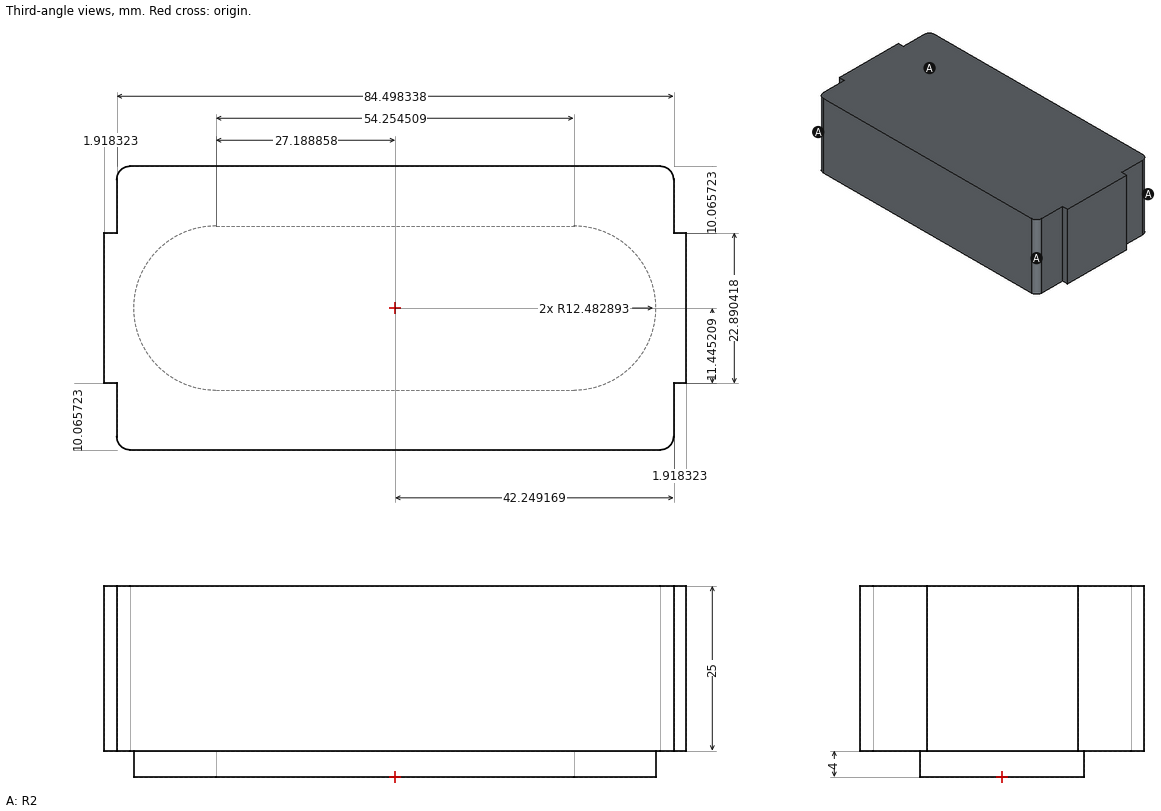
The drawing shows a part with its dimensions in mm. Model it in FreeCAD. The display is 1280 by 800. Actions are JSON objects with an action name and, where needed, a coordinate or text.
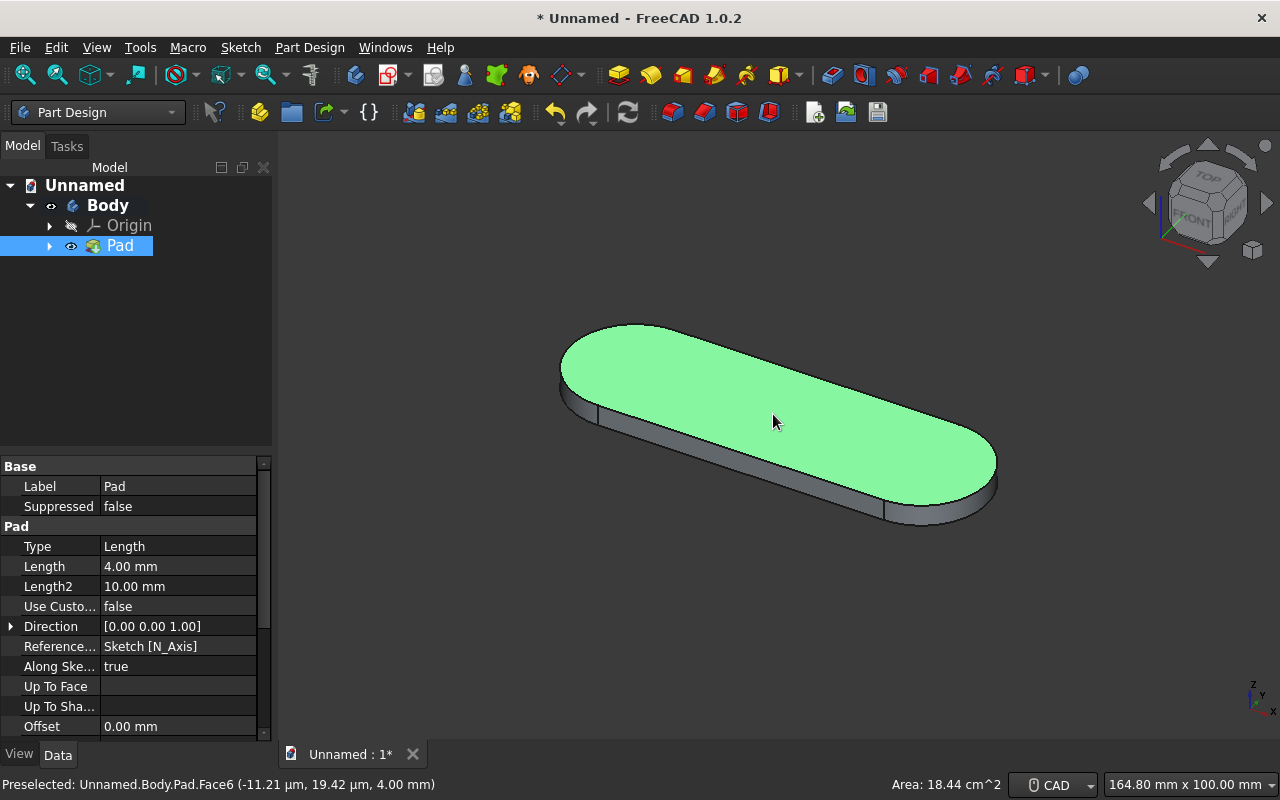
{"action": "left_click", "coordinate": [388, 76]}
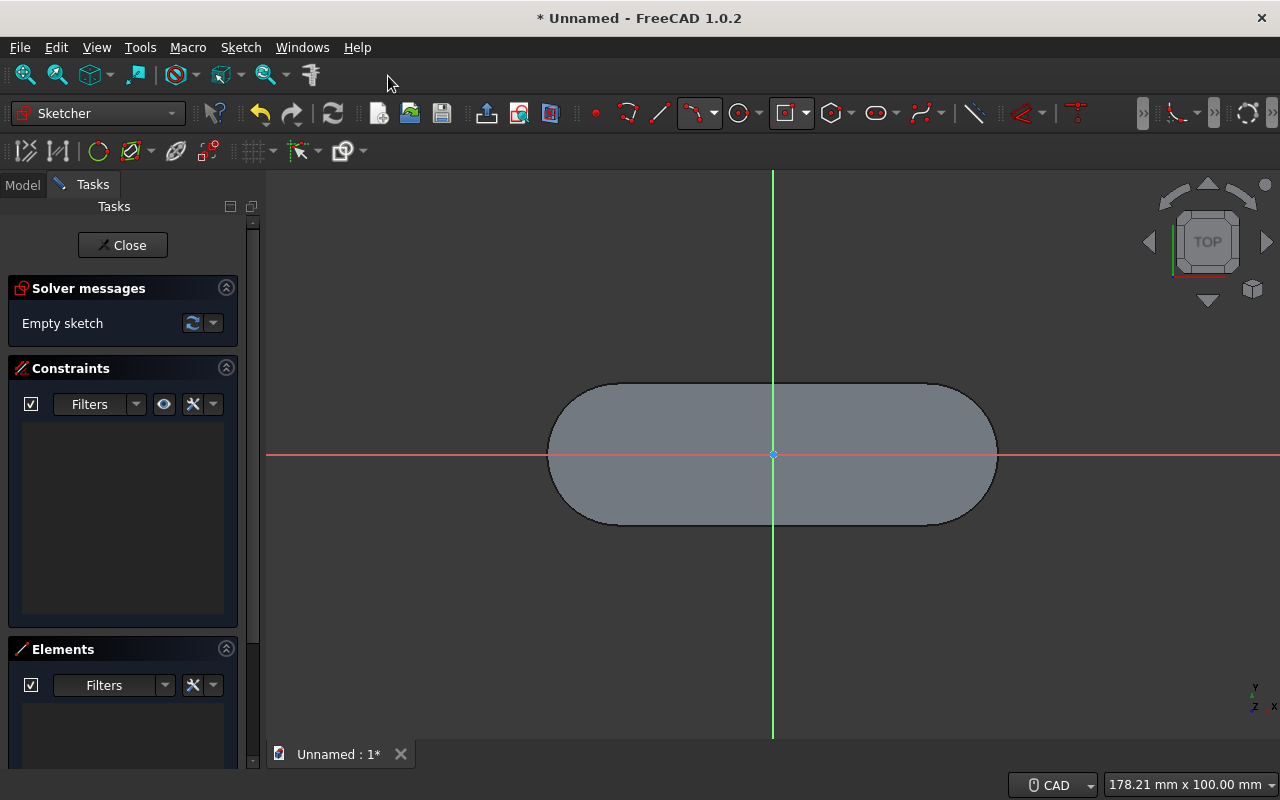
{"action": "left_click", "coordinate": [628, 114]}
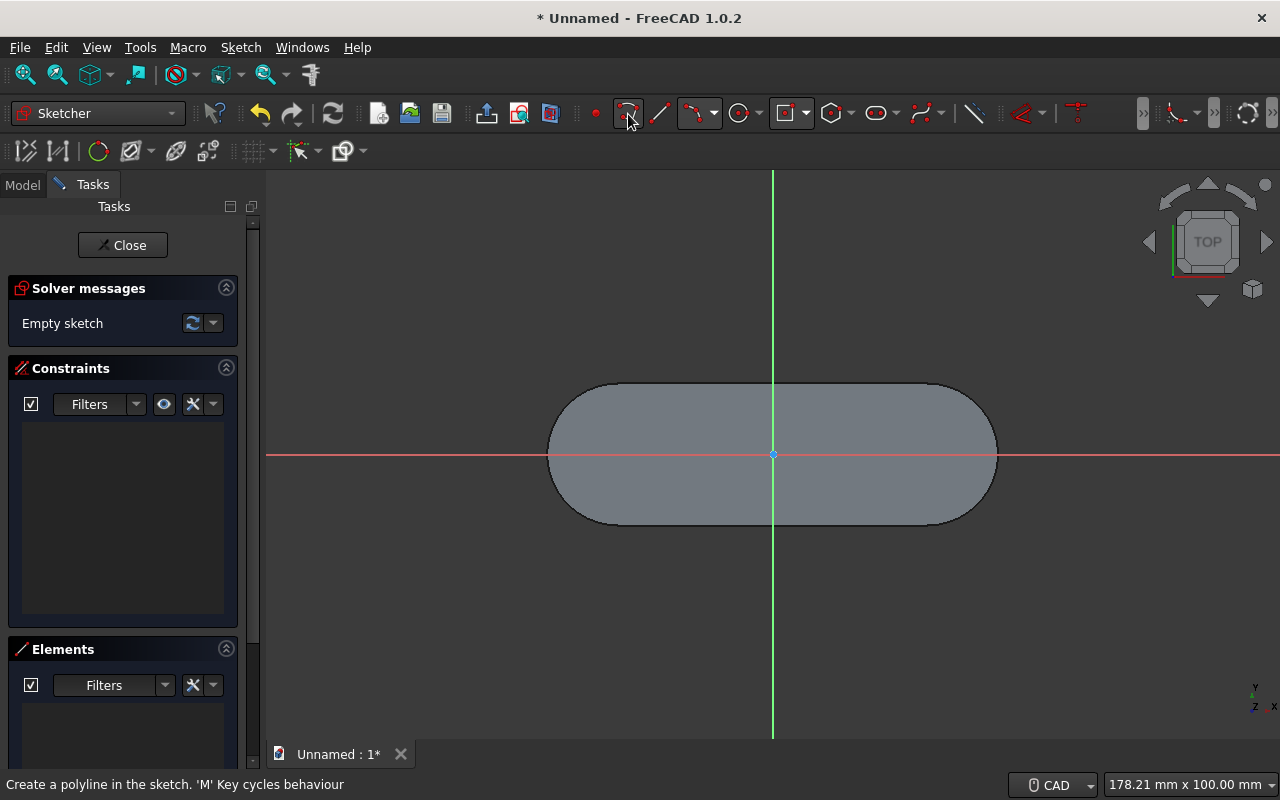
{"action": "left_click", "coordinate": [1013, 520]}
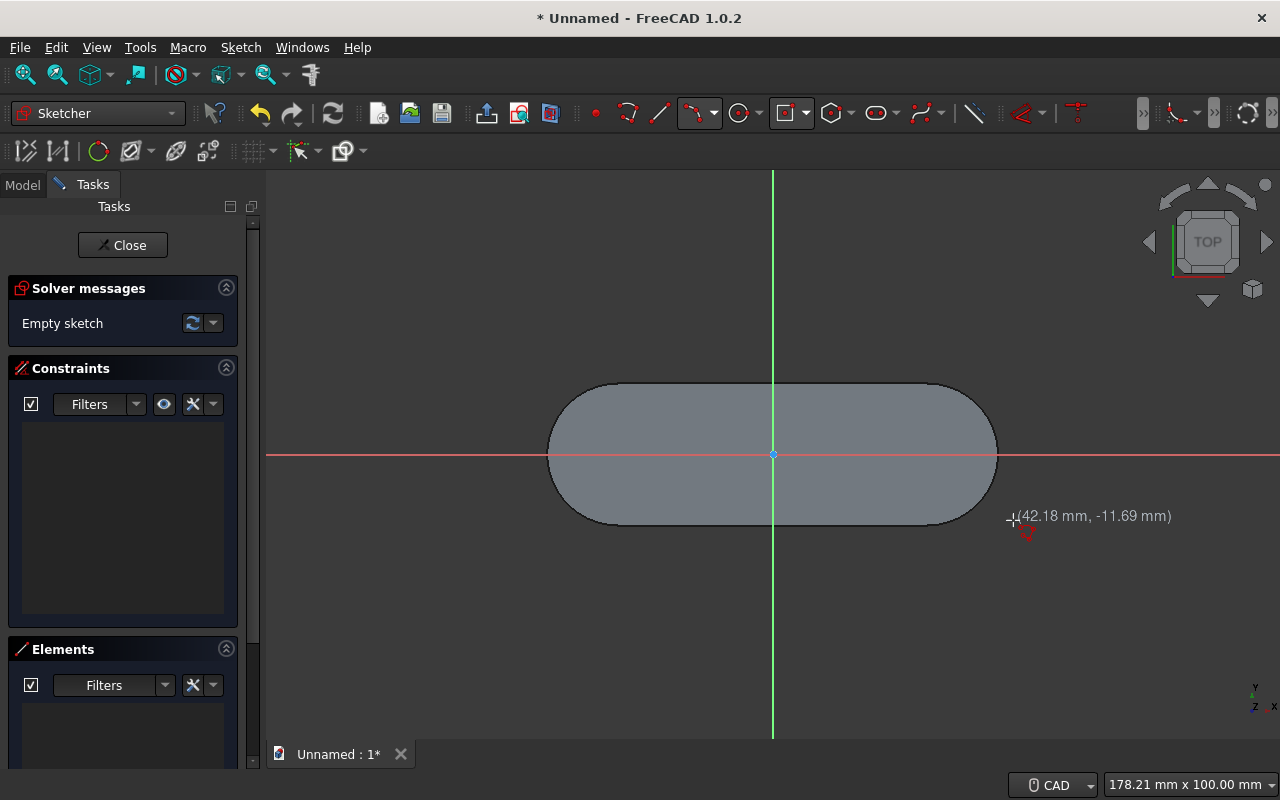
{"action": "scroll", "coordinate": [1024, 520], "scroll_direction": "up", "scroll_amount": 2}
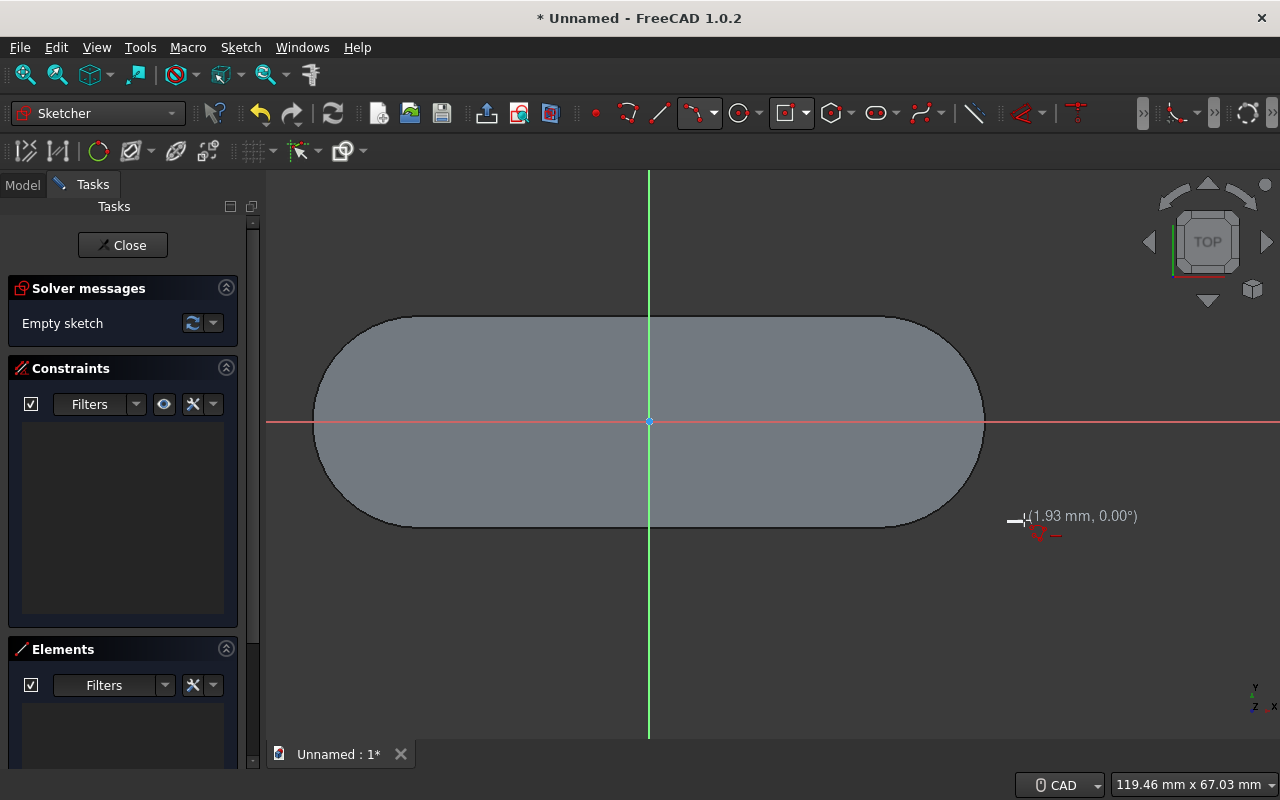
{"action": "left_click", "coordinate": [1024, 520]}
{"action": "left_click", "coordinate": [1024, 325]}
{"action": "left_click", "coordinate": [1008, 325]}
{"action": "left_click", "coordinate": [1008, 239]}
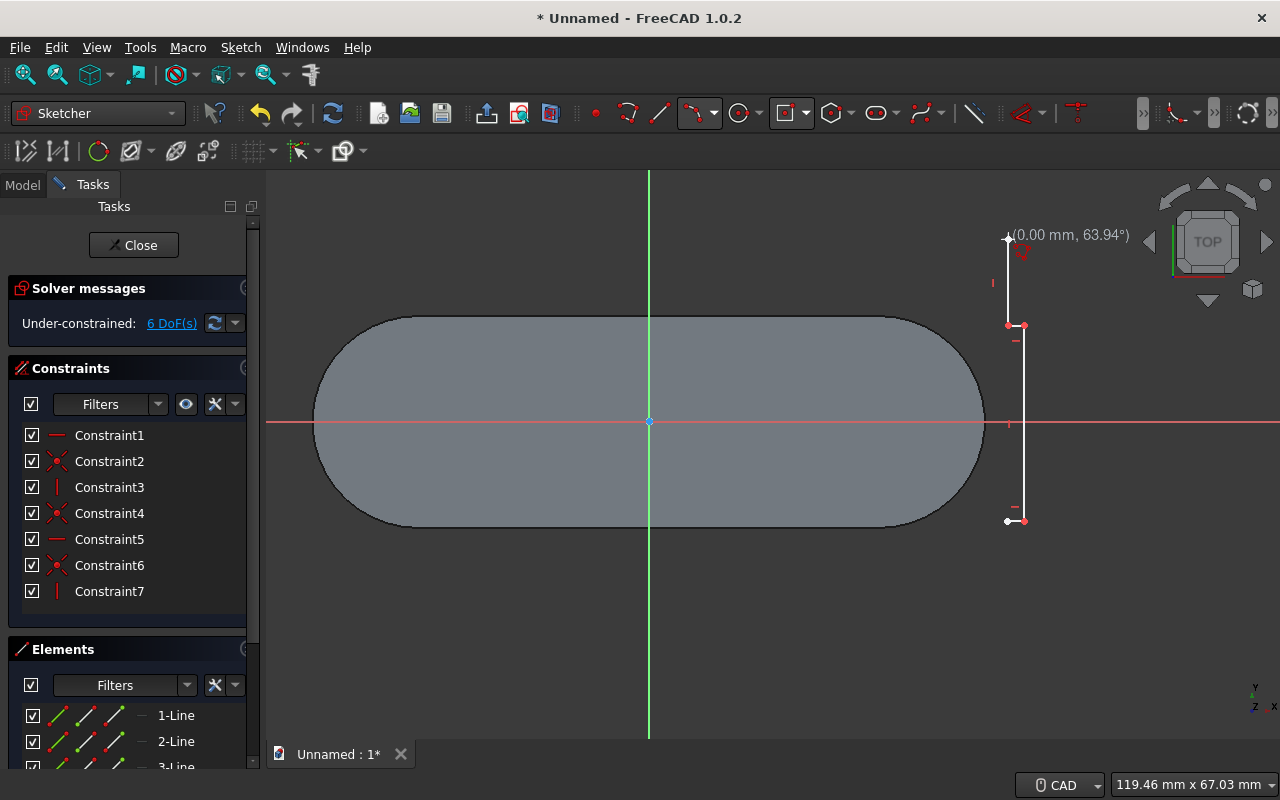
{"action": "scroll", "coordinate": [954, 601], "scroll_direction": "down", "scroll_amount": 1}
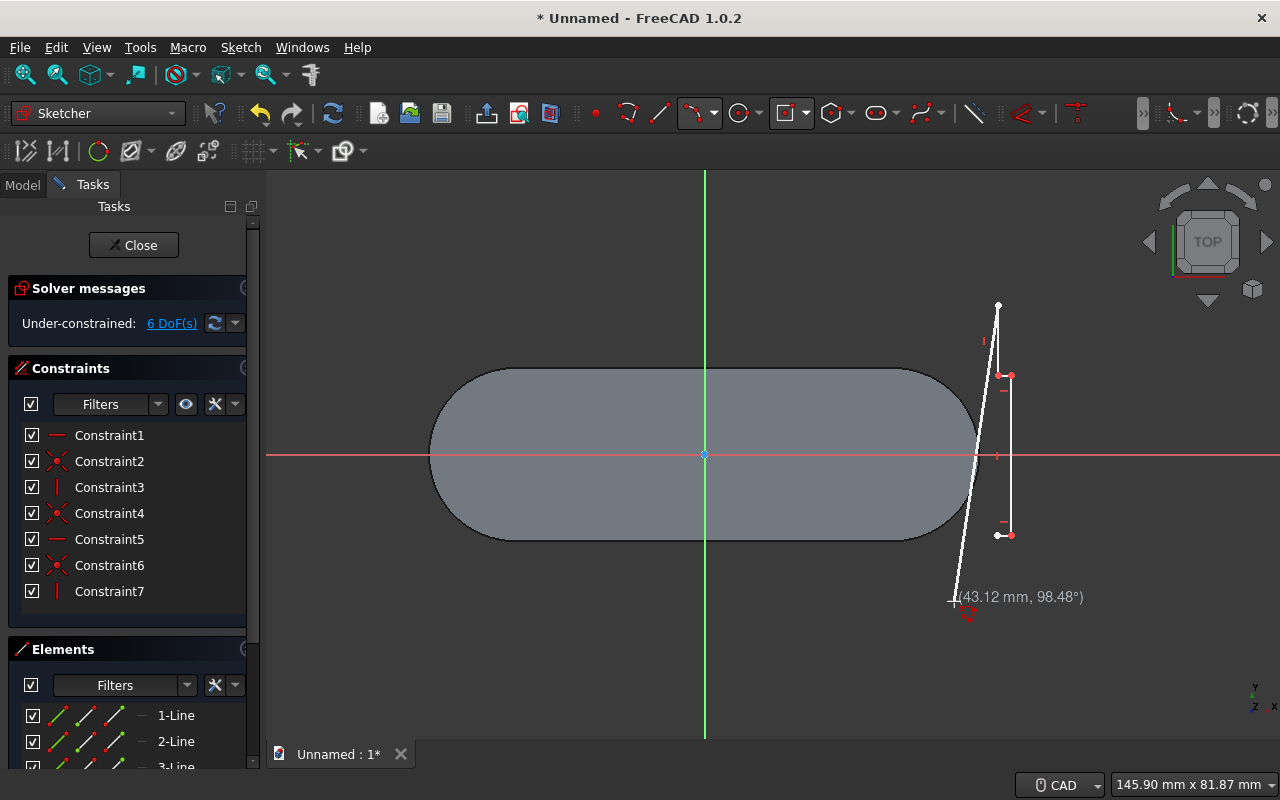
{"action": "left_click", "coordinate": [411, 305]}
{"action": "left_click", "coordinate": [411, 375]}
{"action": "left_click", "coordinate": [398, 375]}
{"action": "left_click", "coordinate": [398, 534]}
{"action": "left_click", "coordinate": [411, 534]}
{"action": "left_click", "coordinate": [411, 604]}
{"action": "left_click", "coordinate": [998, 604]}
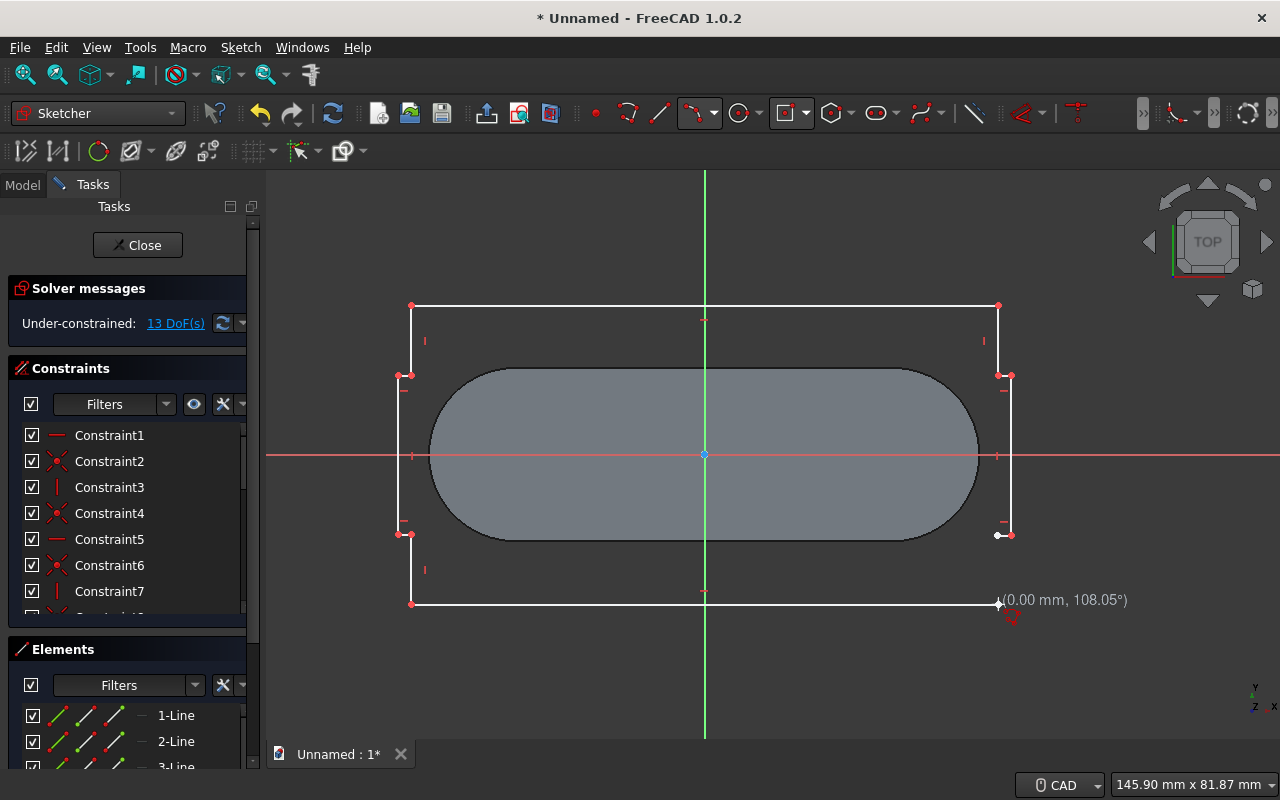
{"action": "scroll", "coordinate": [998, 534], "scroll_direction": "up", "scroll_amount": 5}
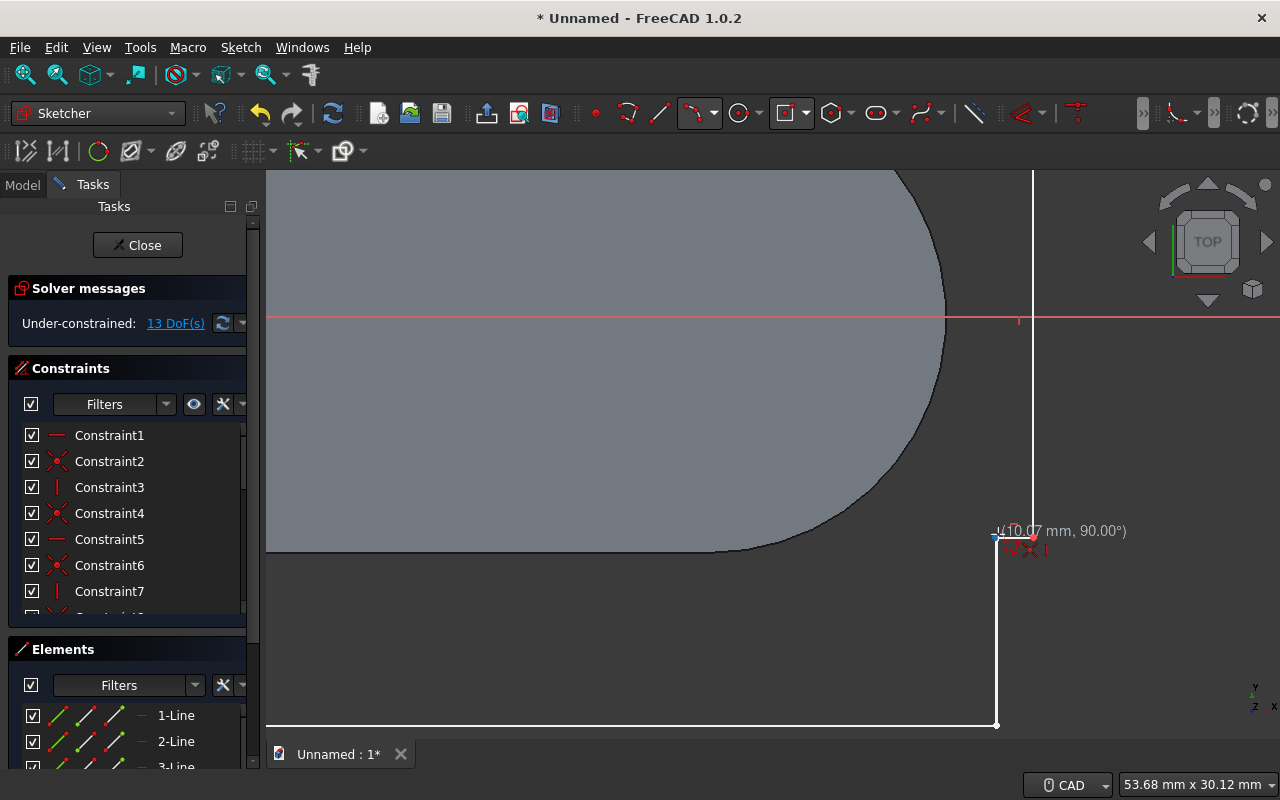
{"action": "left_click", "coordinate": [996, 538]}
{"action": "key", "text": "Escape"}
{"action": "key", "text": "Escape"}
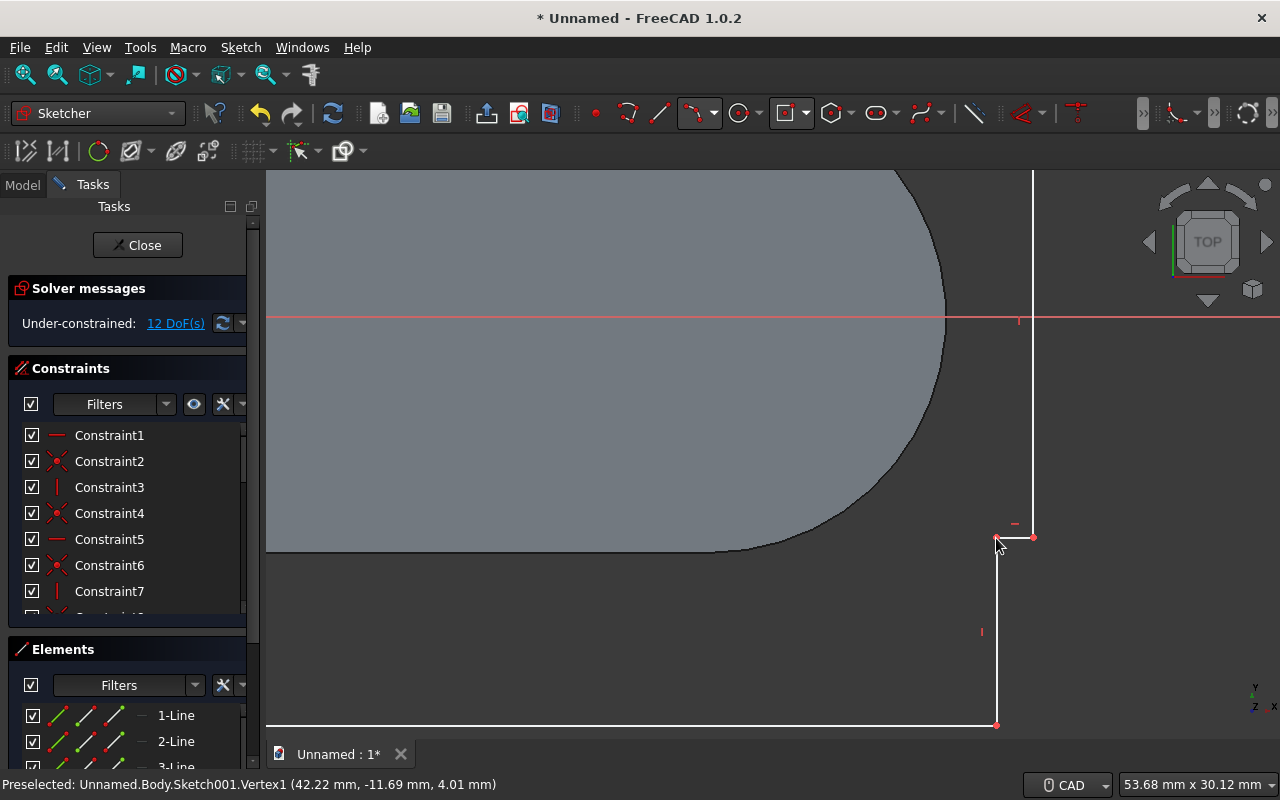
{"action": "left_click", "coordinate": [1022, 114]}